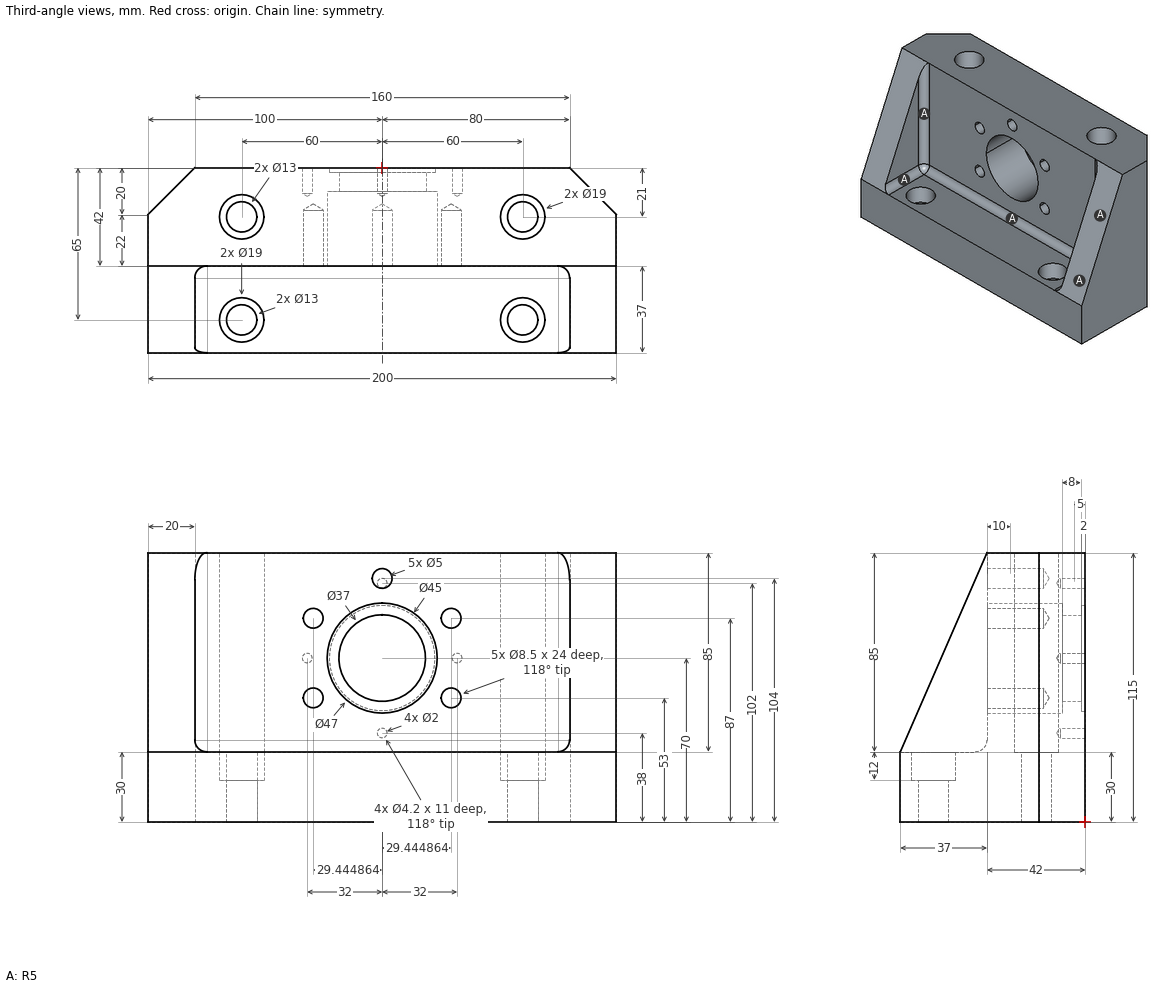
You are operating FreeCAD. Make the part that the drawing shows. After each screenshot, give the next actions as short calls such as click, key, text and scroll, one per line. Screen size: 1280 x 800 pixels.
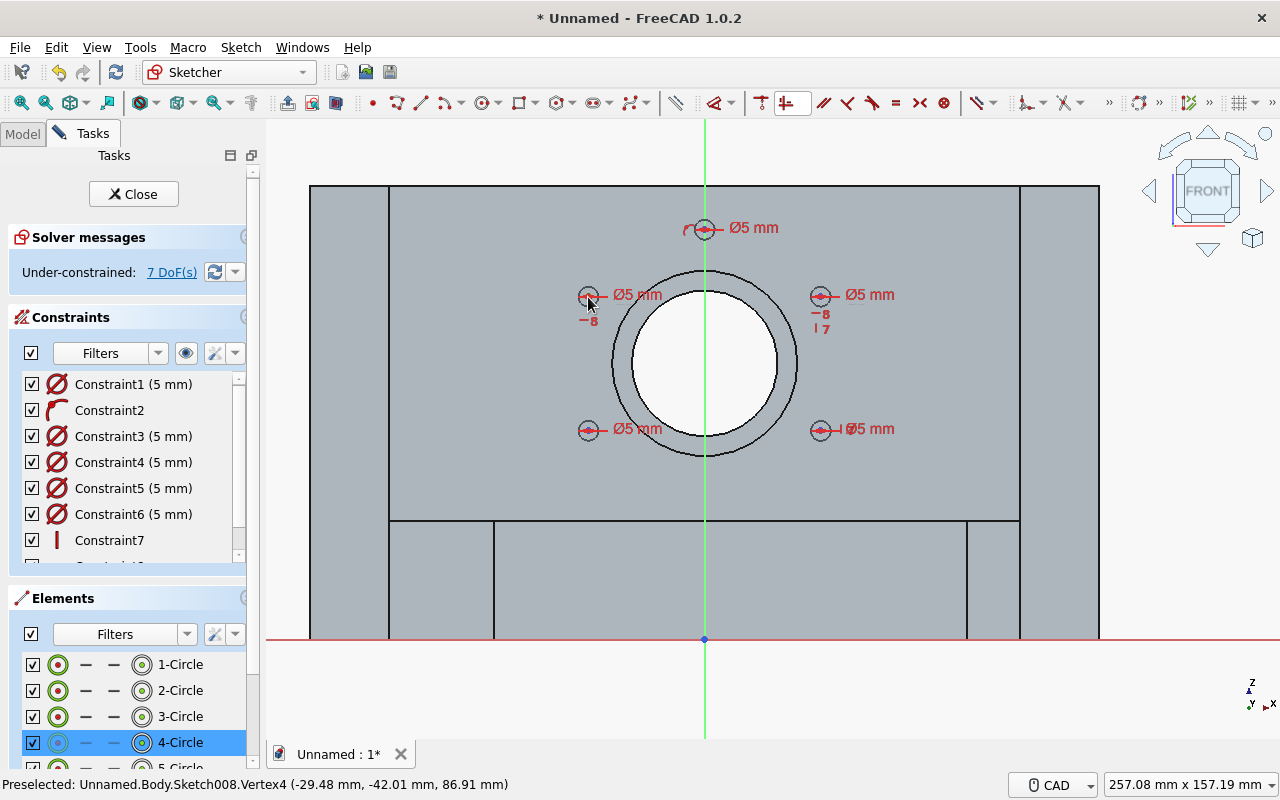
click(588, 431)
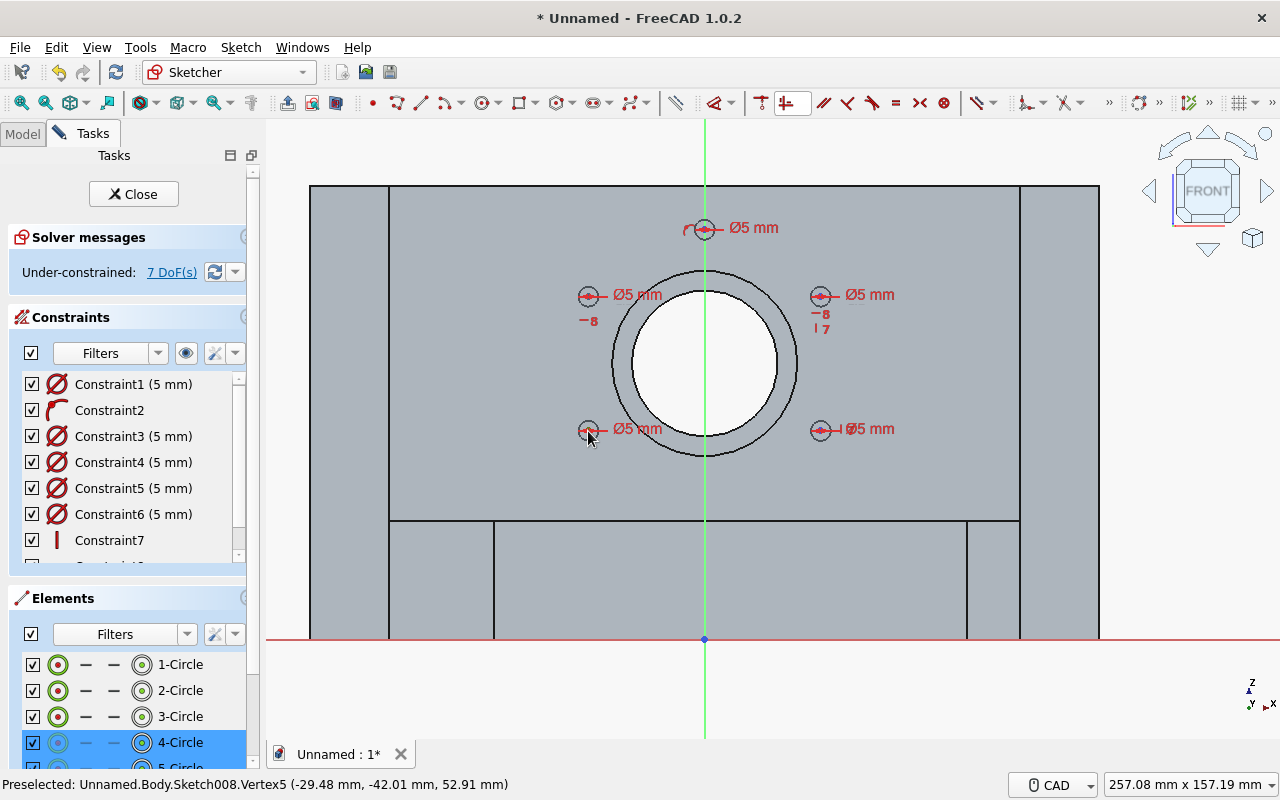
key(v)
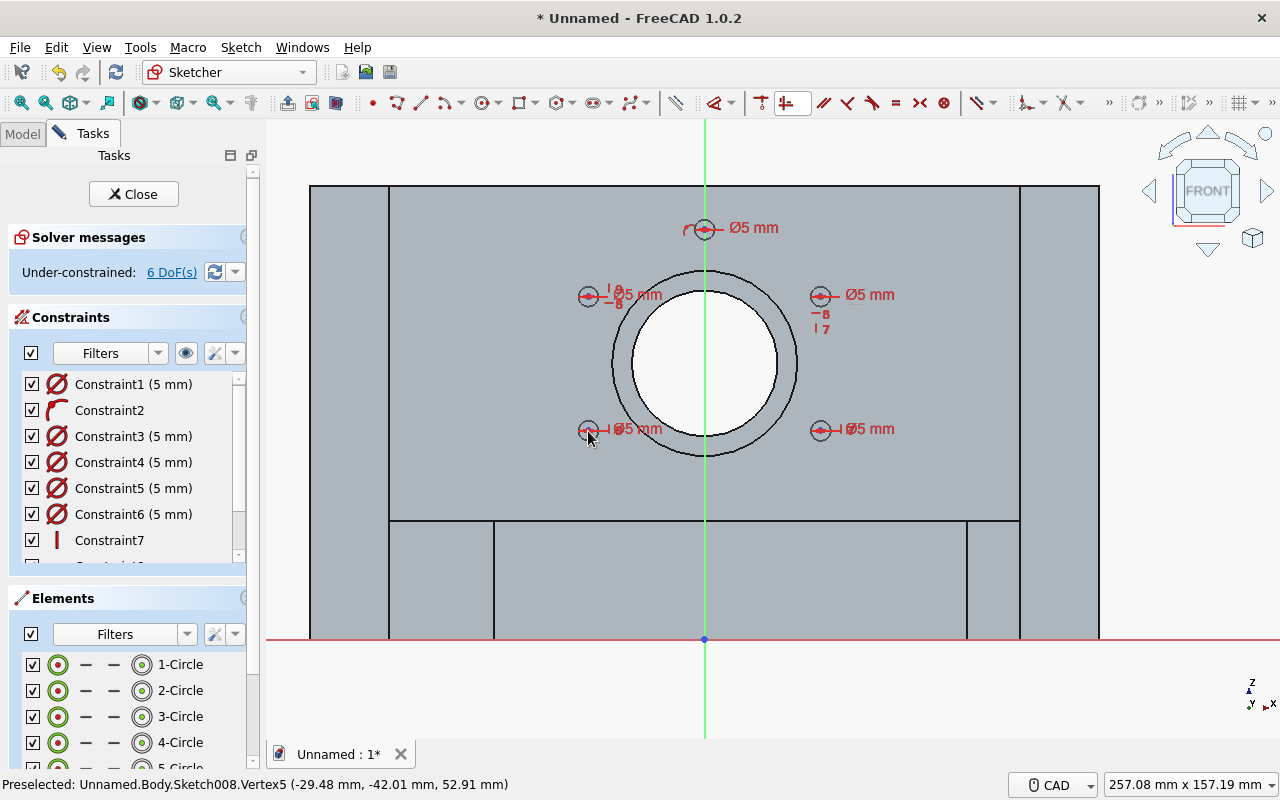
click(821, 431)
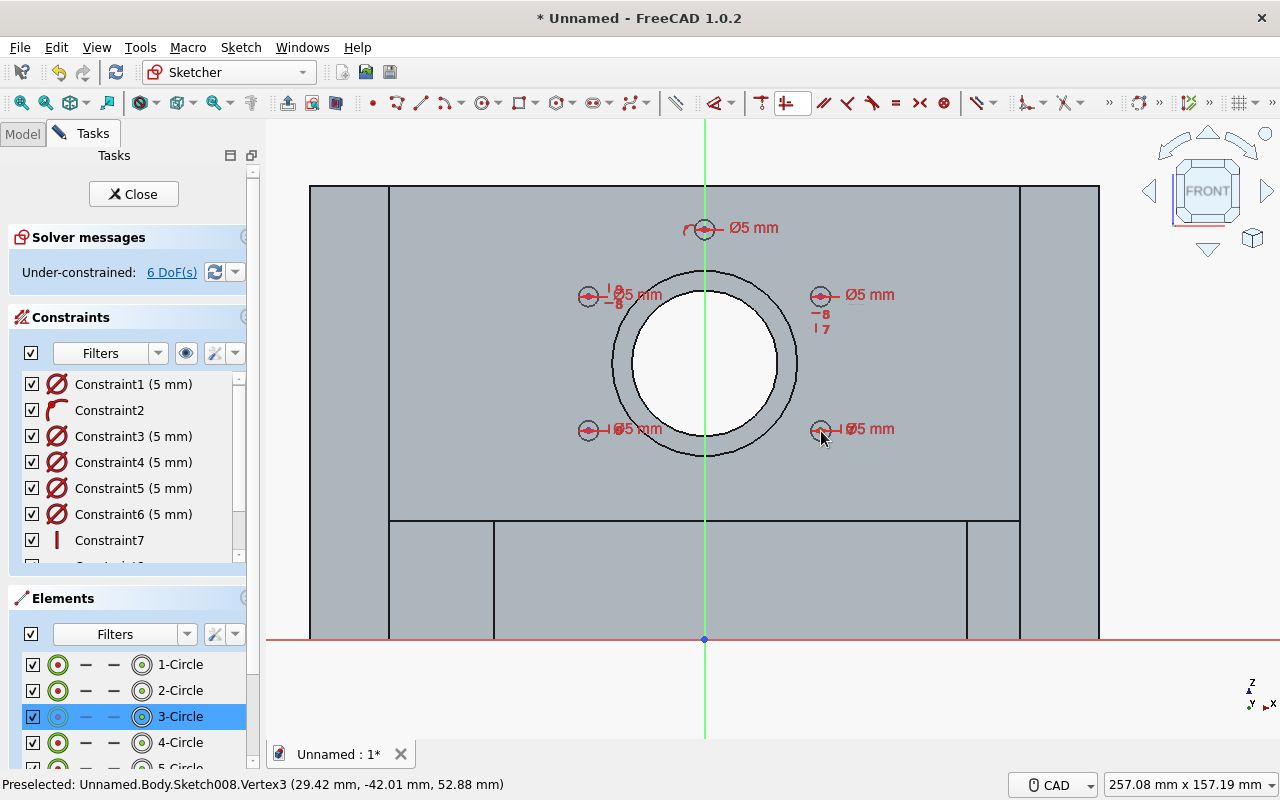
click(588, 431)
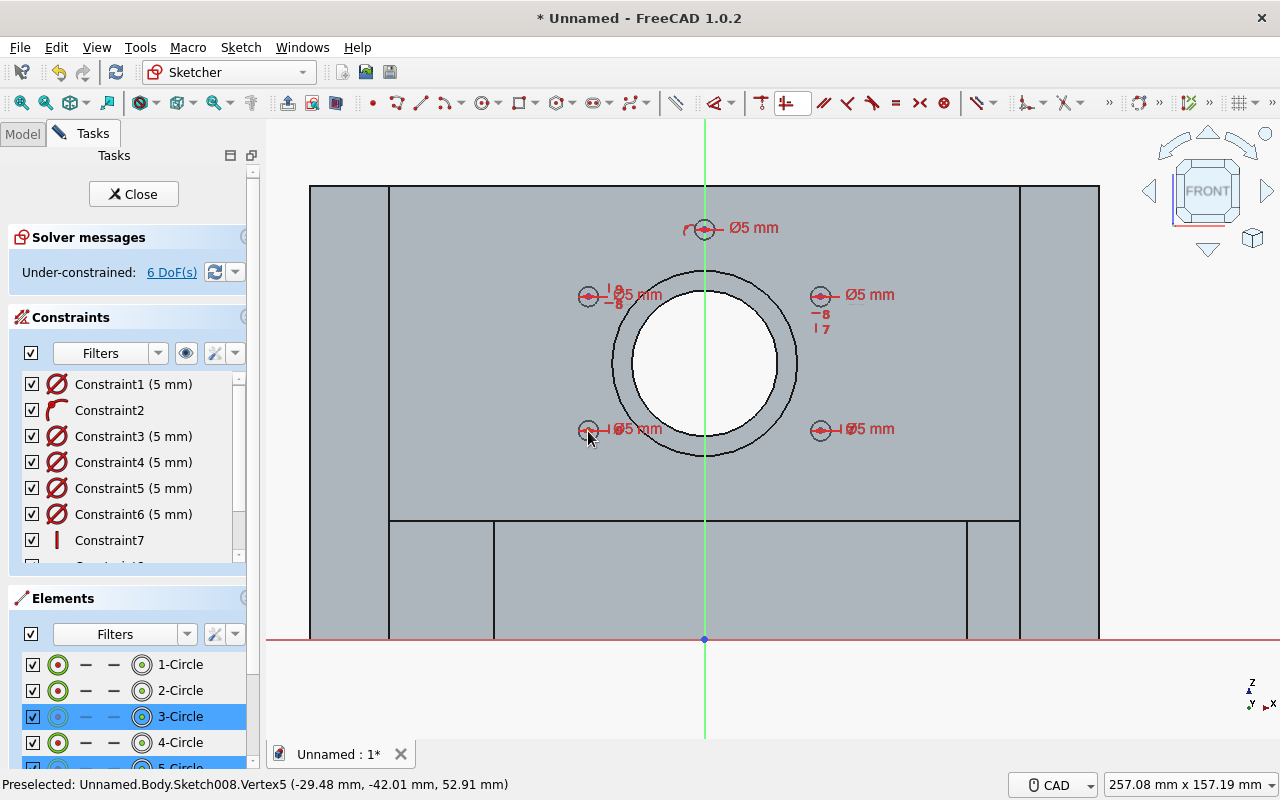
key(h)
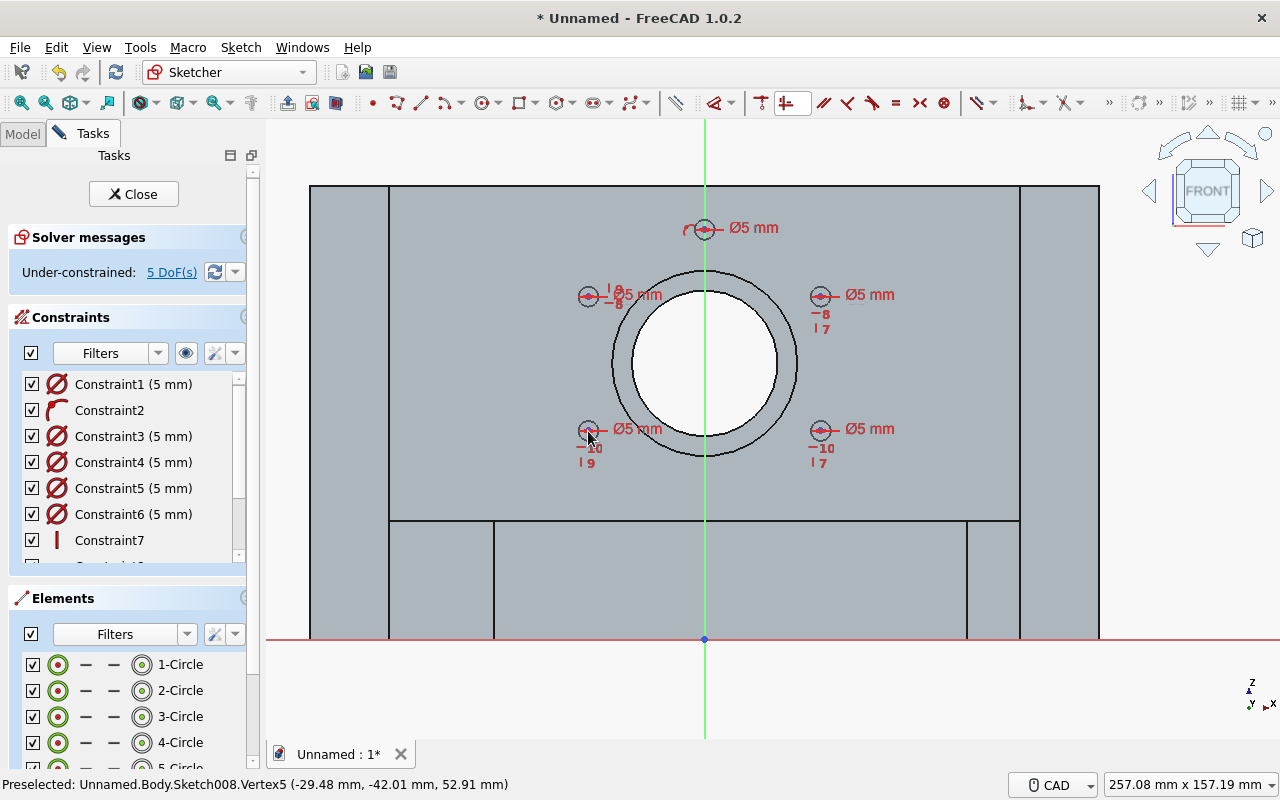
click(714, 104)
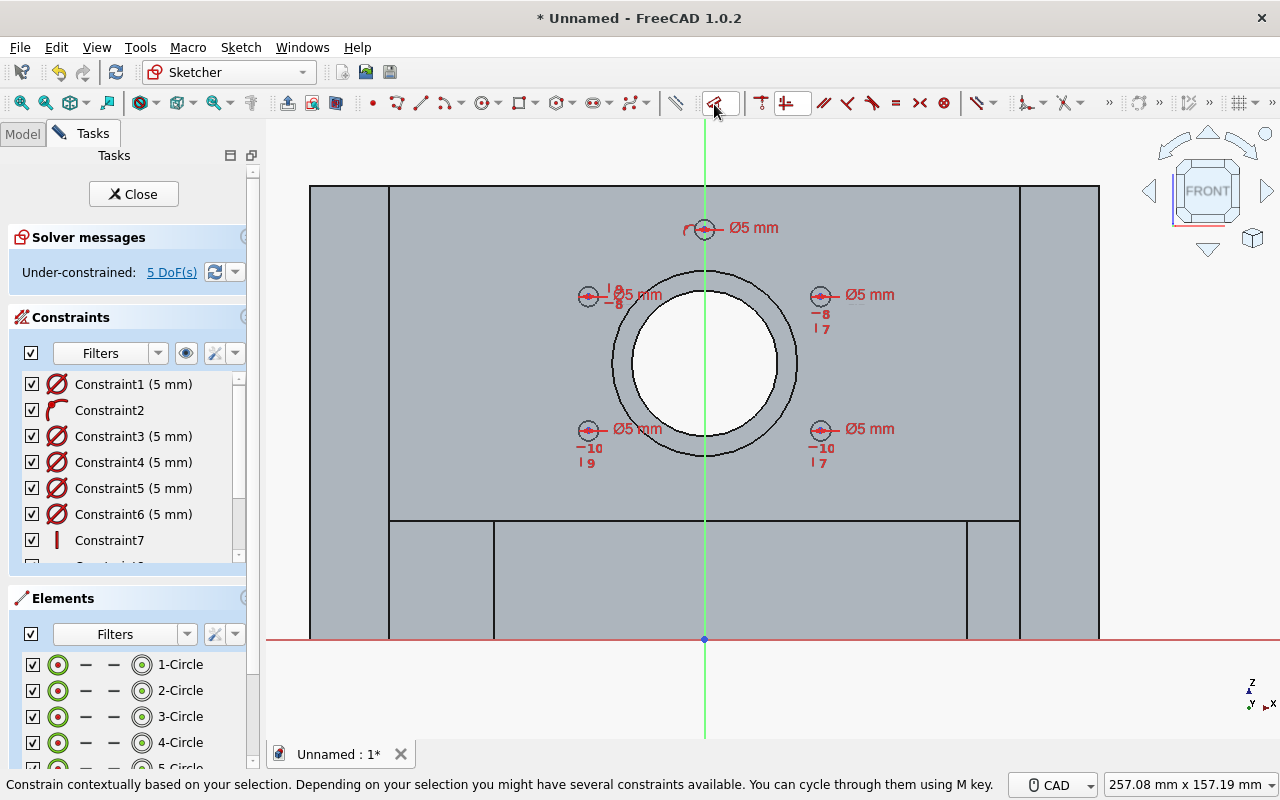
click(821, 297)
click(855, 468)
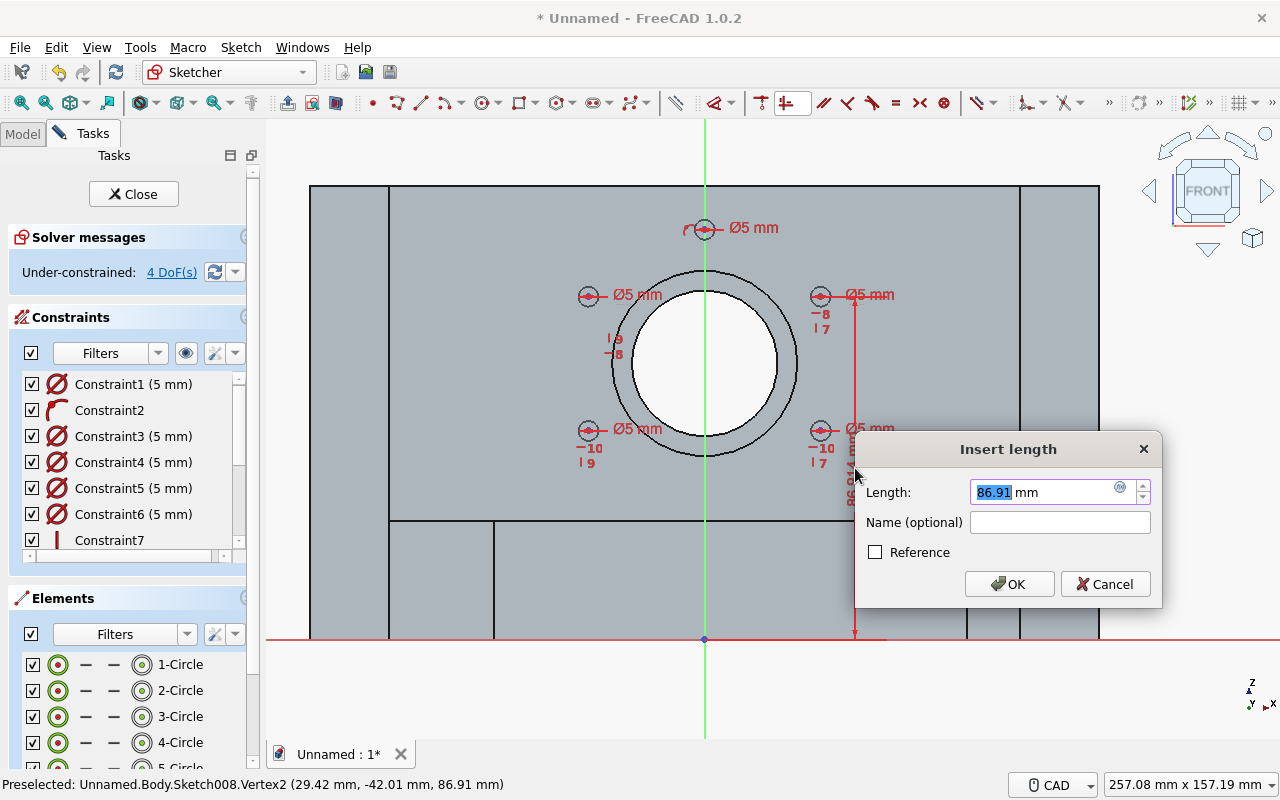
text(87)
key(Return)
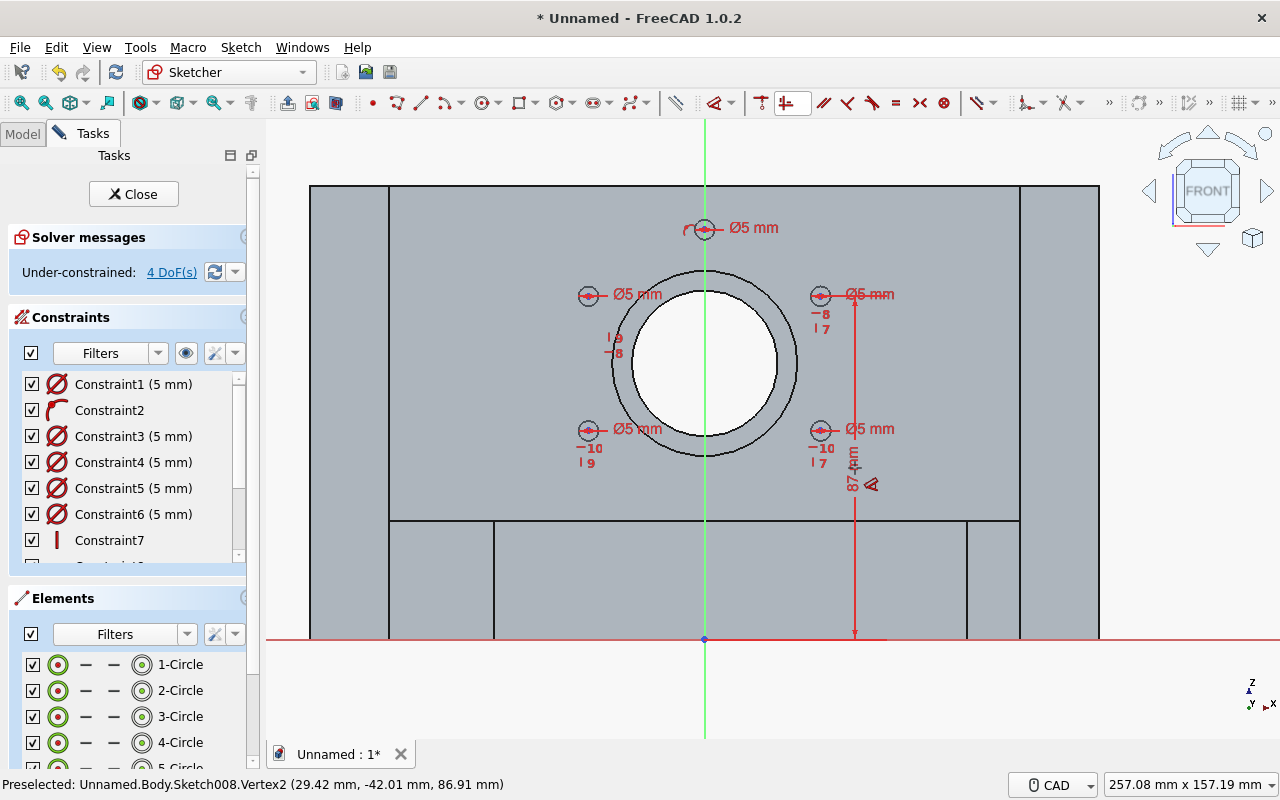
click(821, 431)
click(855, 535)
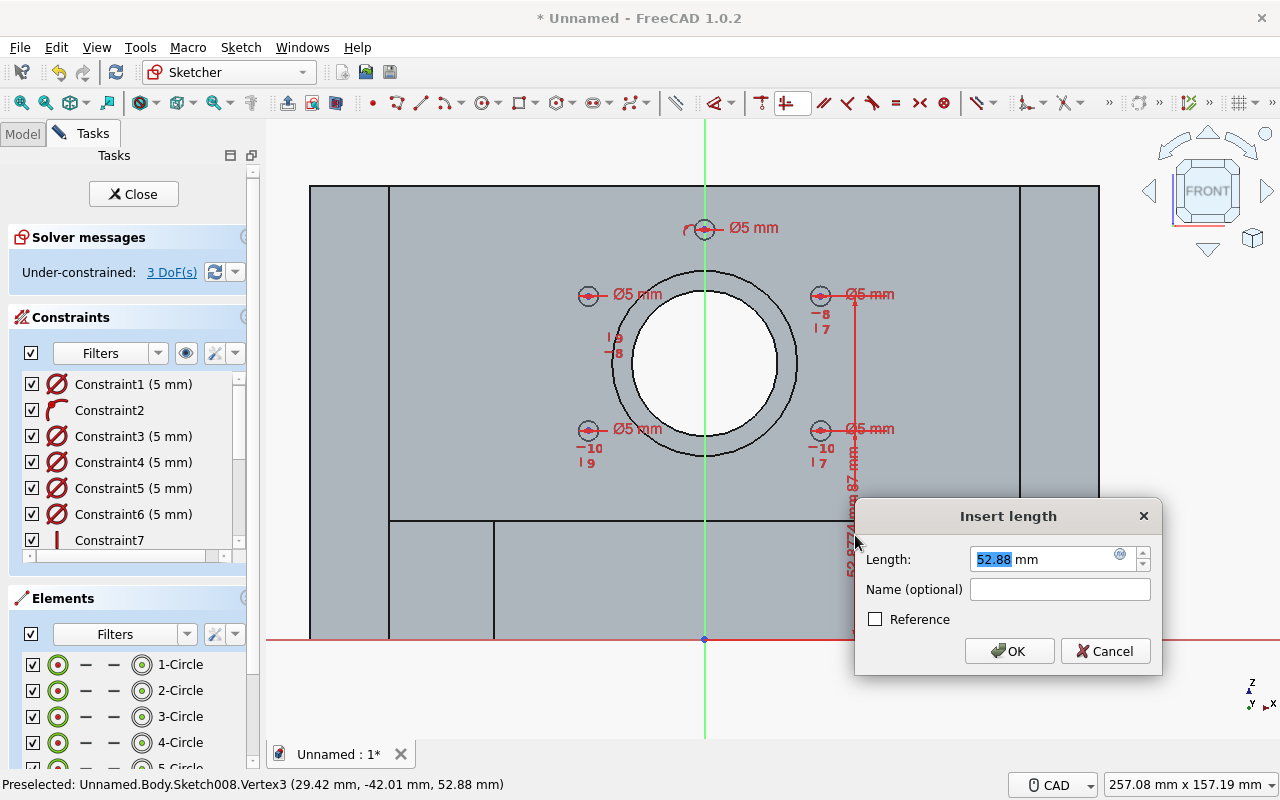
text(53)
key(Return)